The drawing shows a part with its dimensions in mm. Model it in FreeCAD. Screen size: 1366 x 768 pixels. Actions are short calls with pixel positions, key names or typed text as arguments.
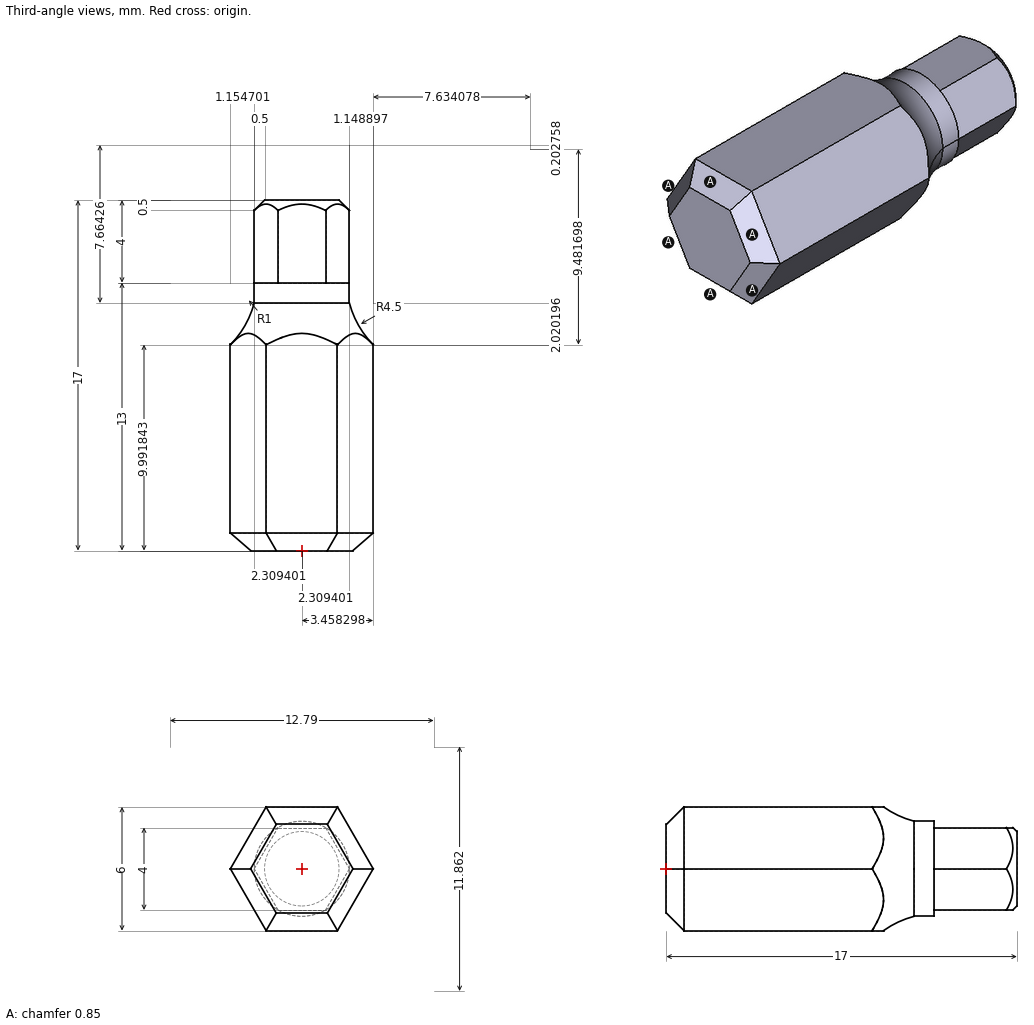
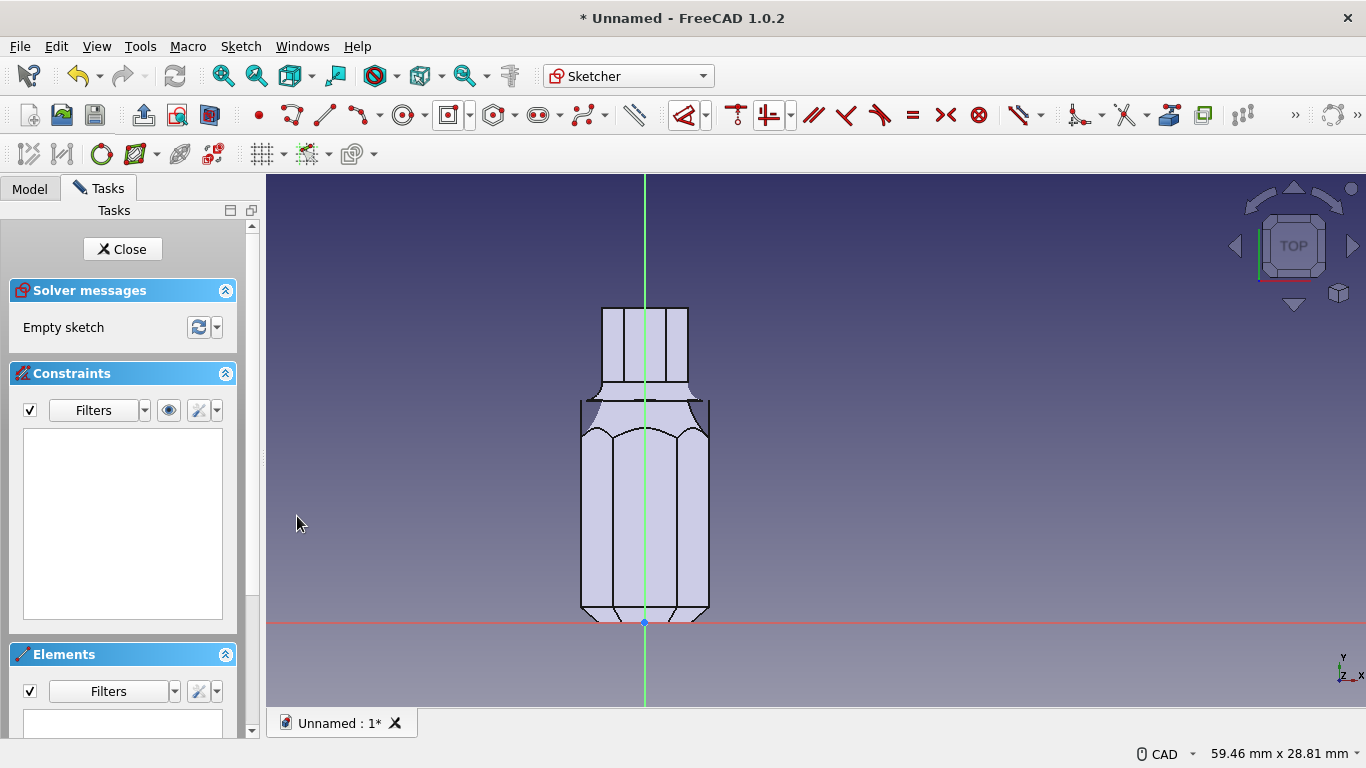
click(292, 116)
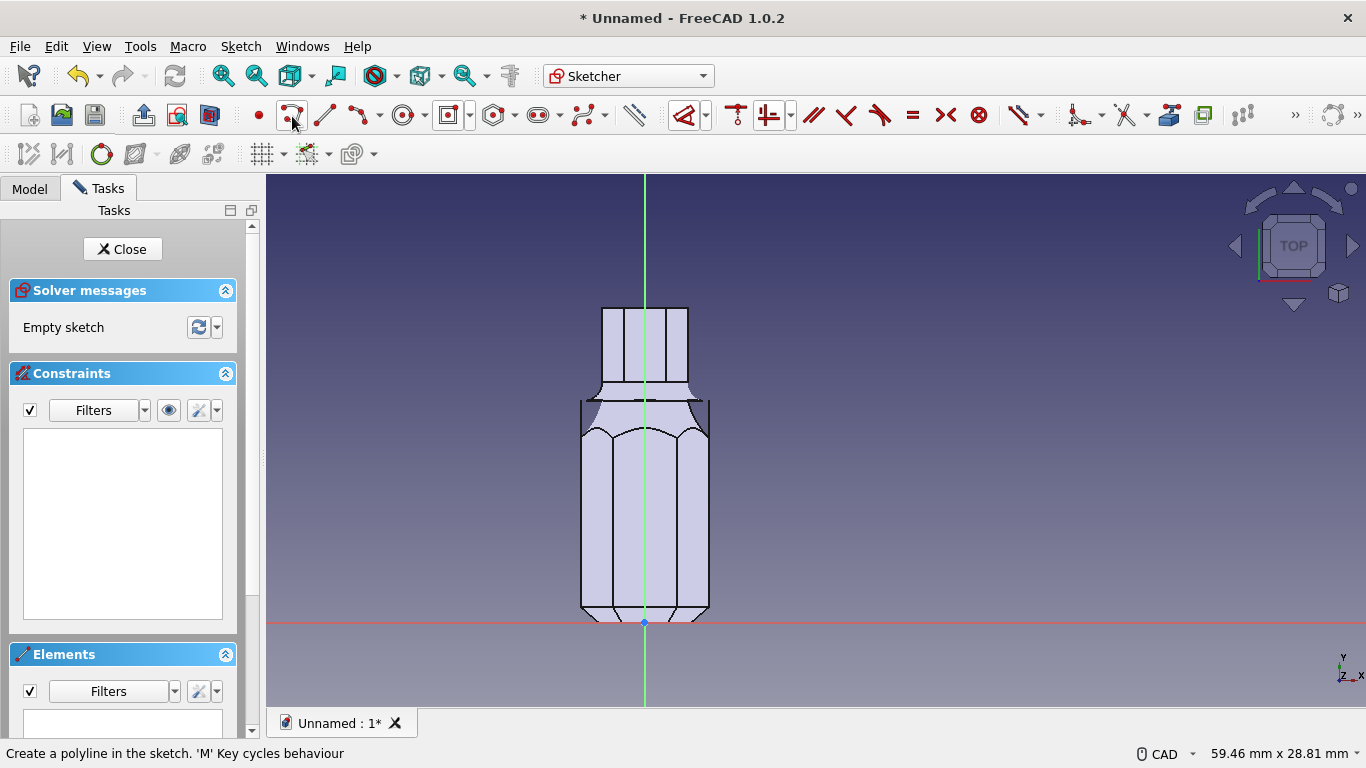
click(709, 438)
click(850, 263)
click(688, 254)
click(688, 401)
right_click(688, 401)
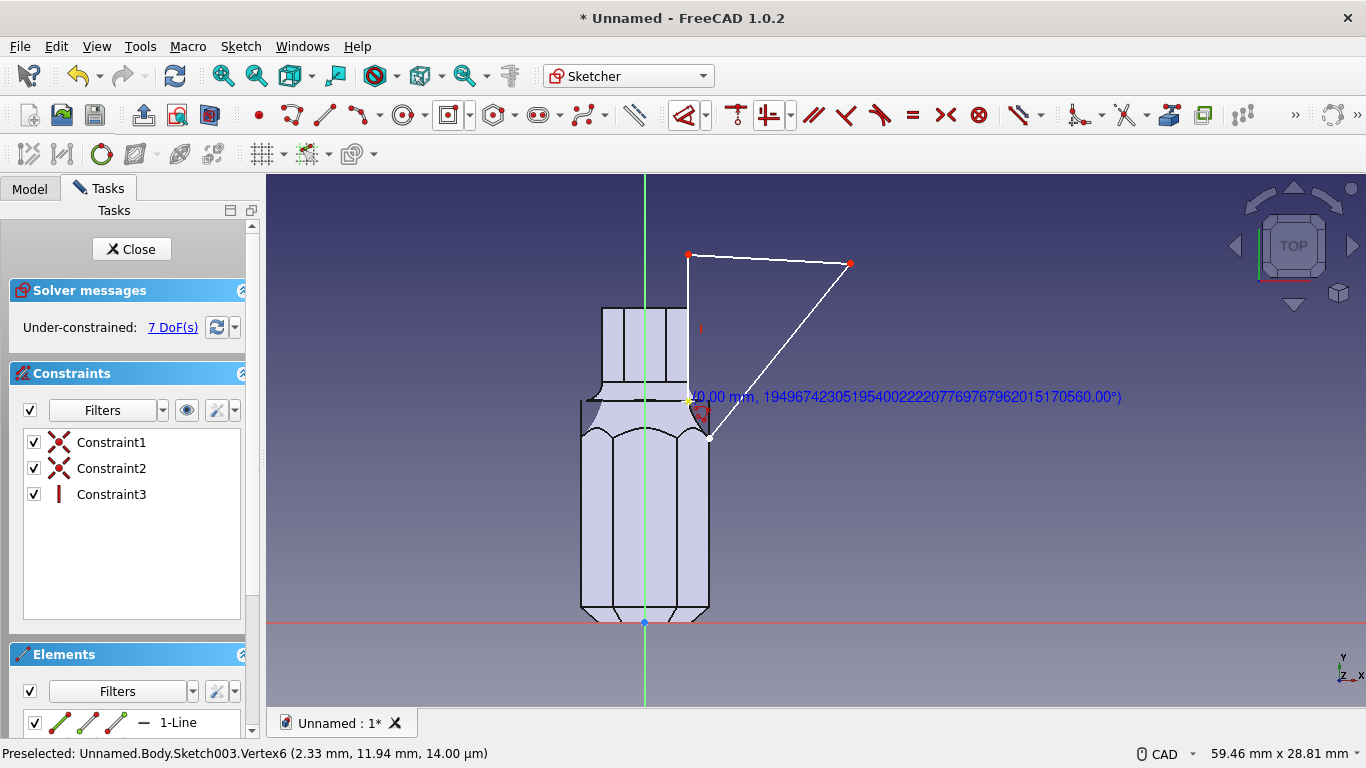
click(358, 116)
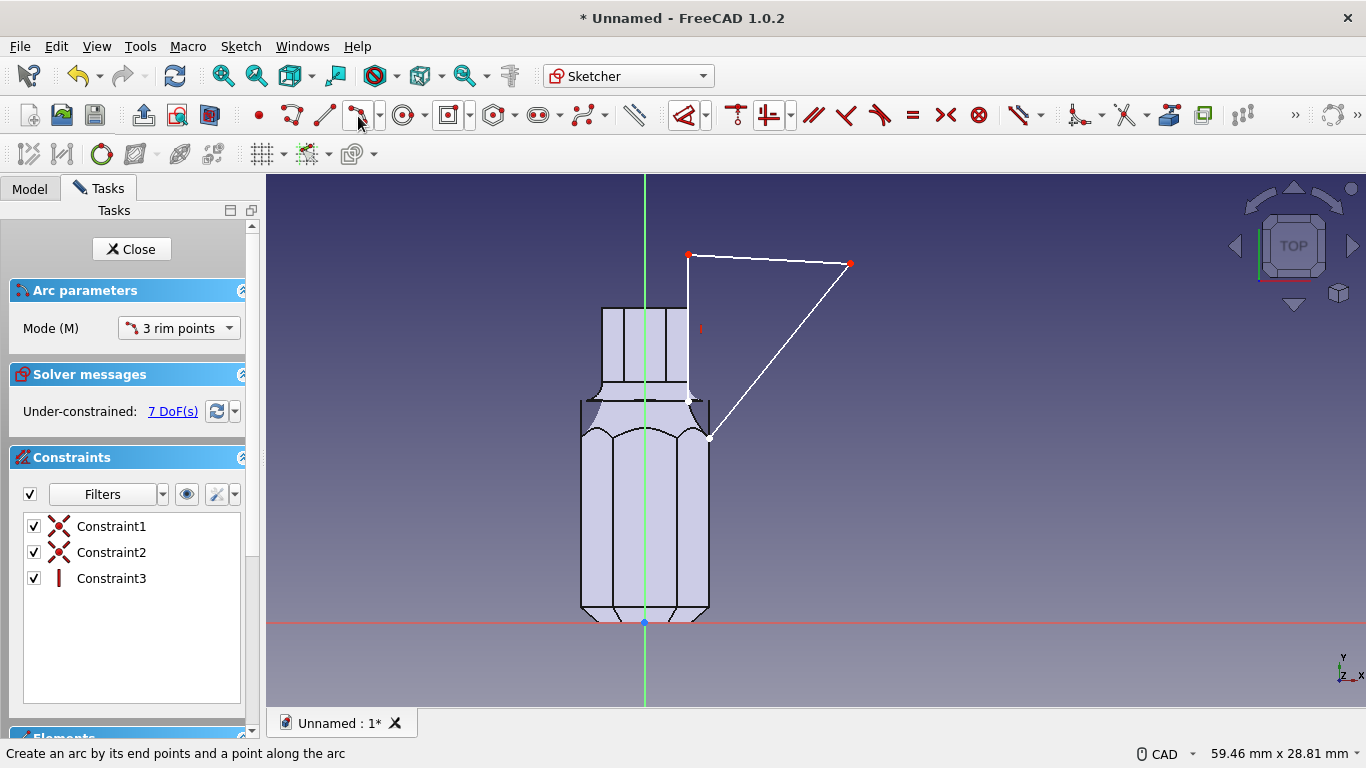
click(688, 402)
click(709, 439)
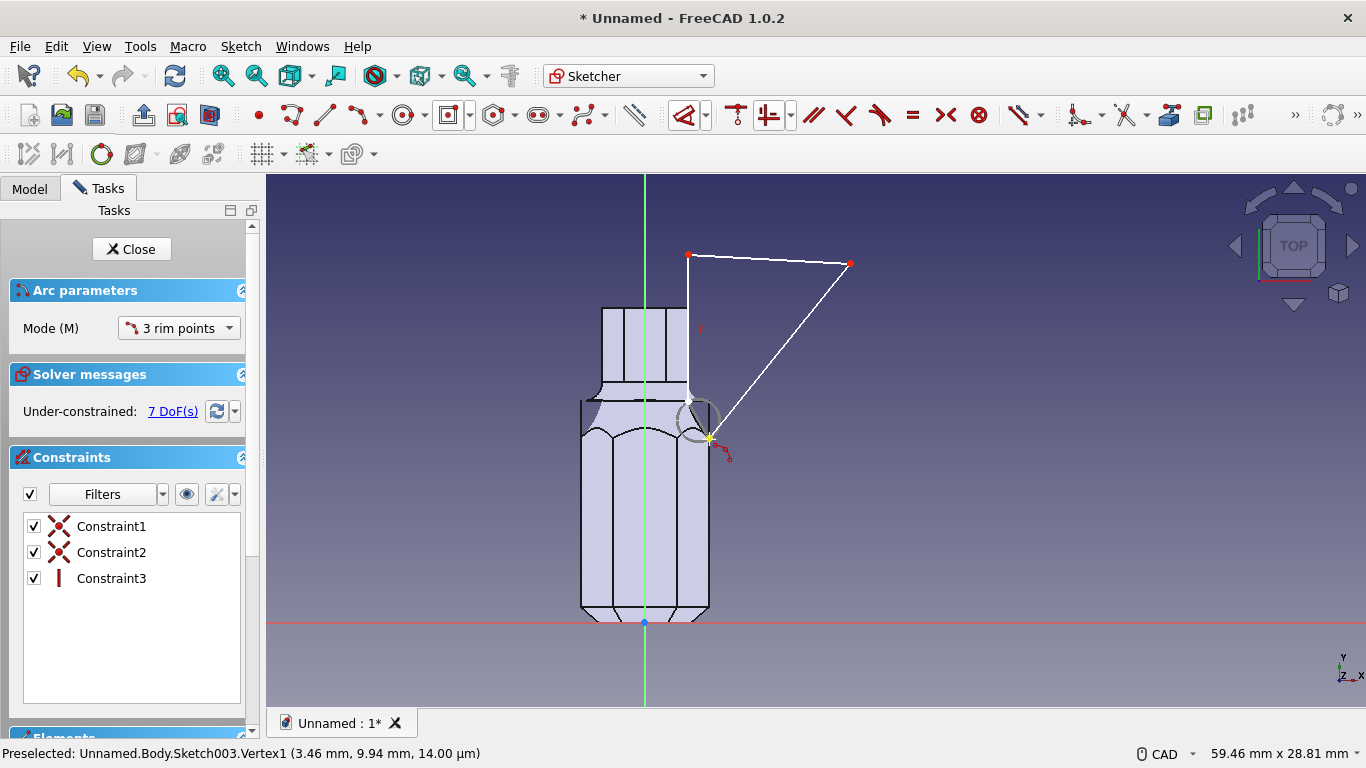
scroll(696, 421, up, 9)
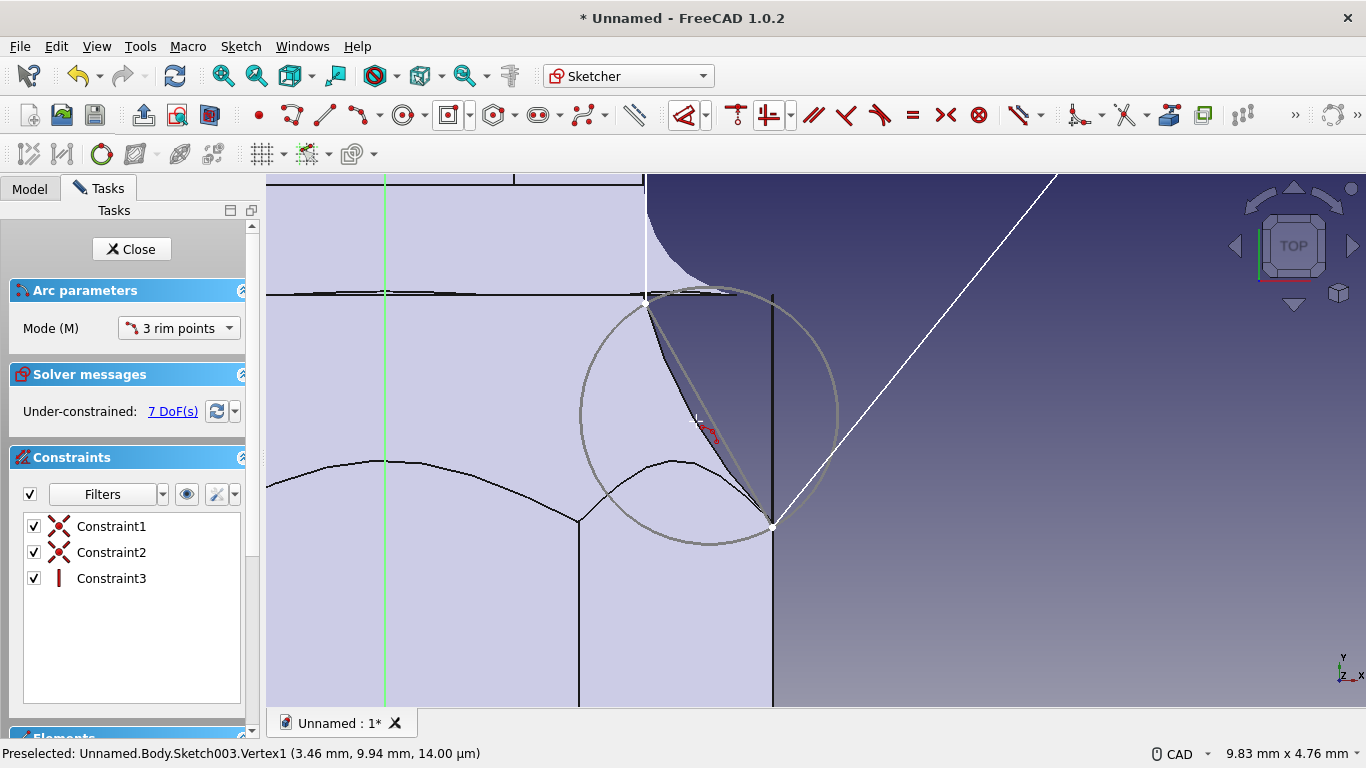
click(693, 417)
key(Escape)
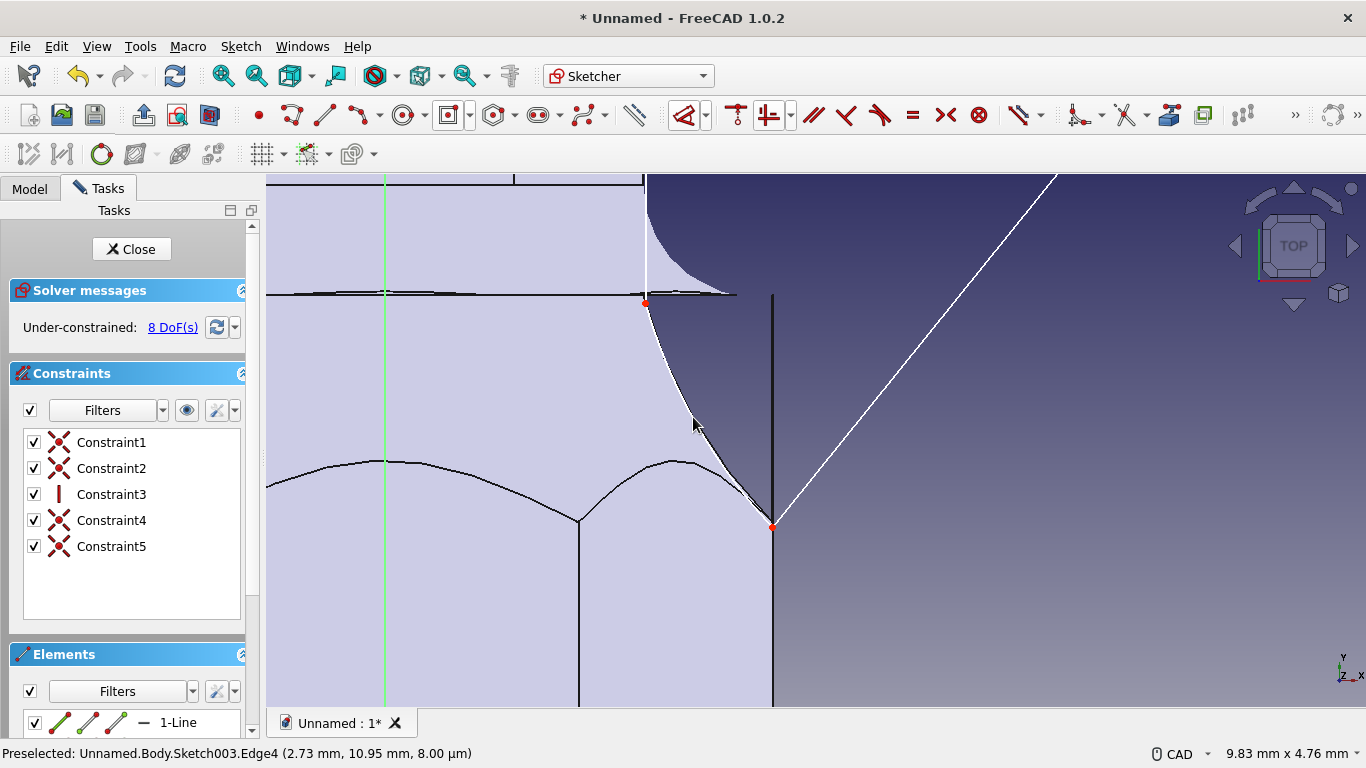
scroll(696, 421, down, 9)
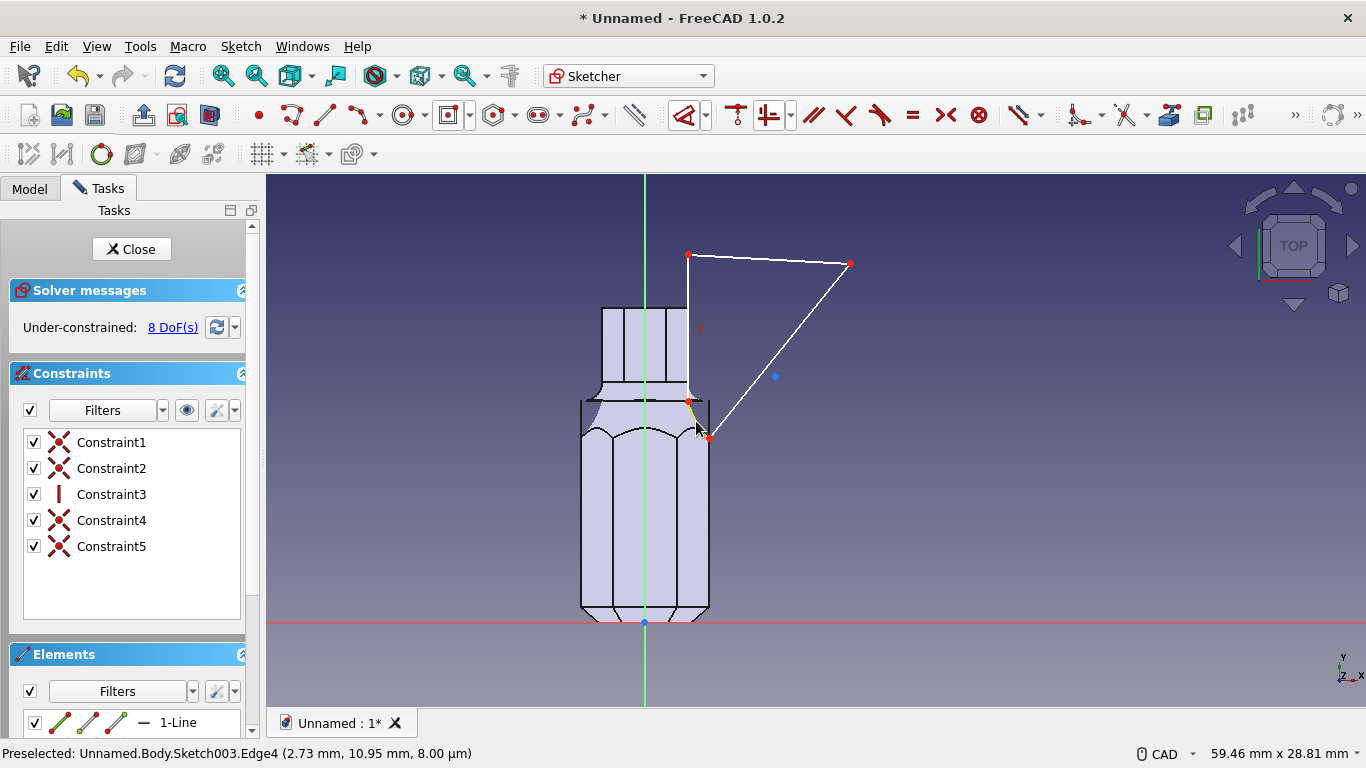
click(692, 414)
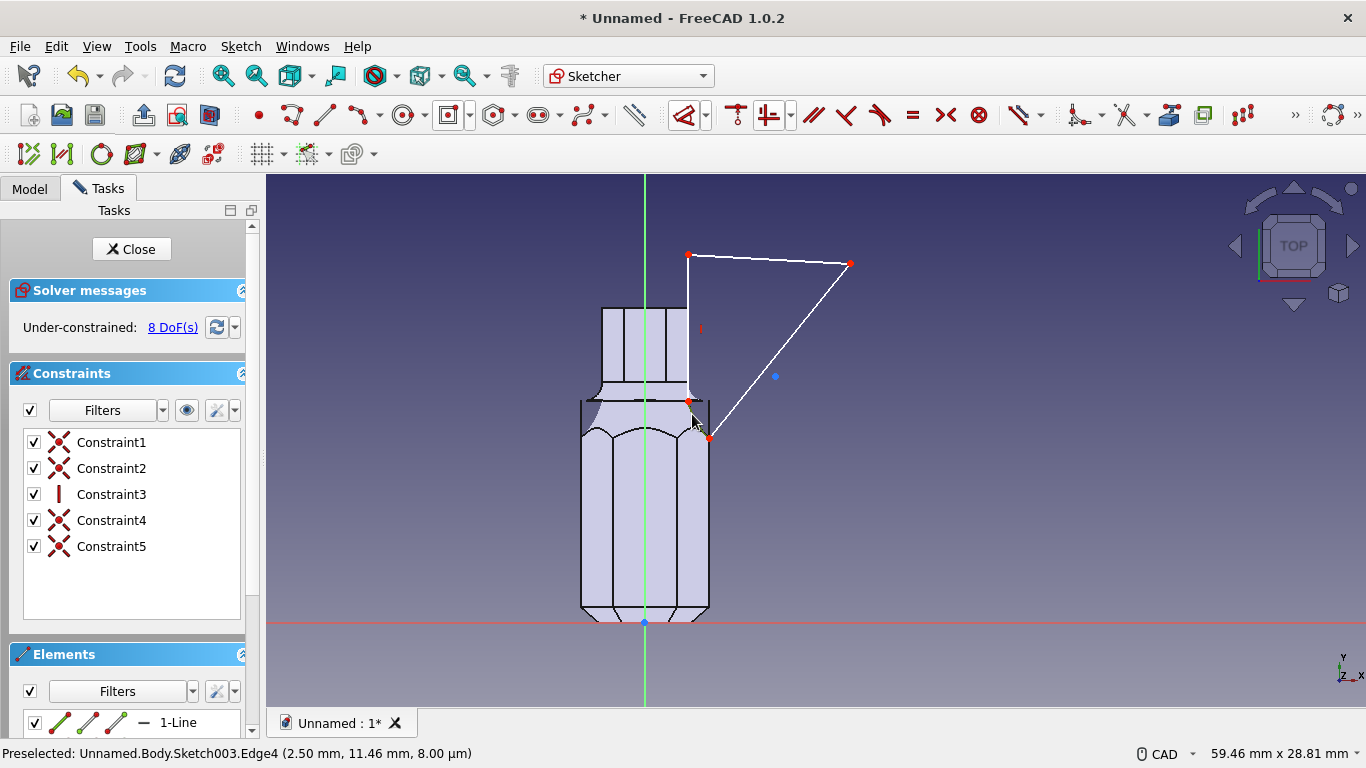
click(706, 116)